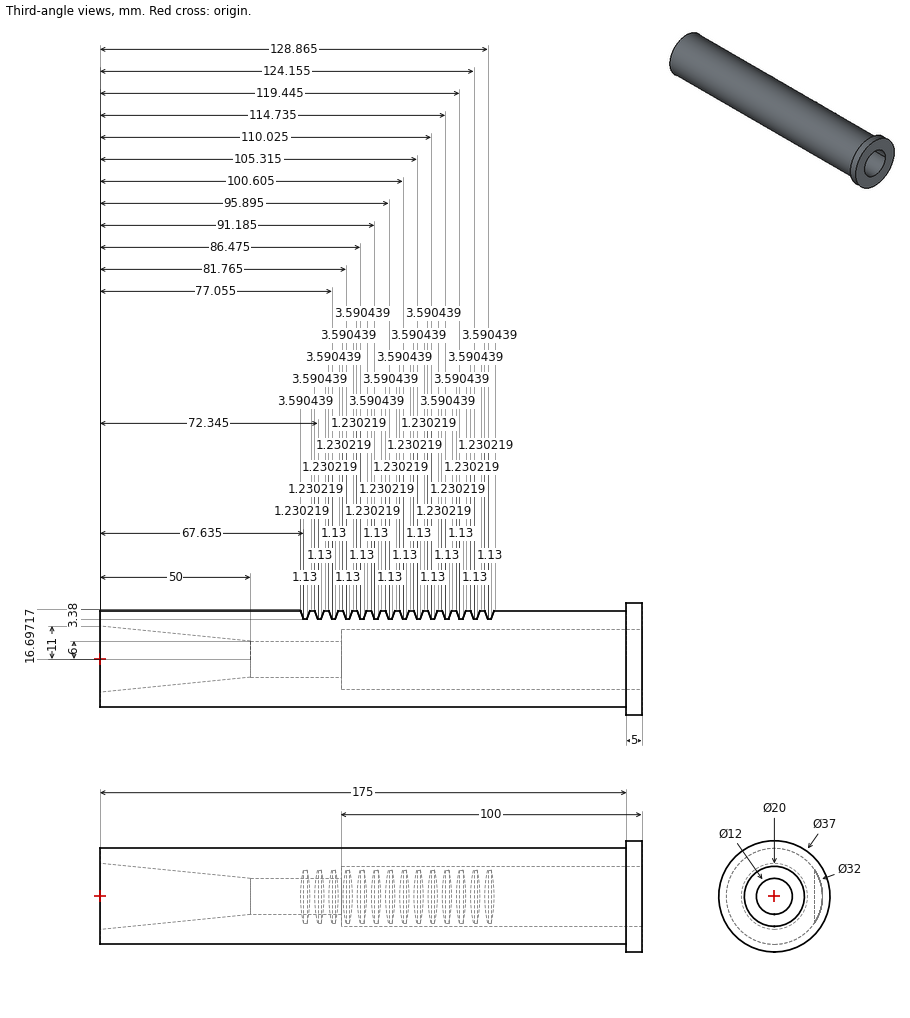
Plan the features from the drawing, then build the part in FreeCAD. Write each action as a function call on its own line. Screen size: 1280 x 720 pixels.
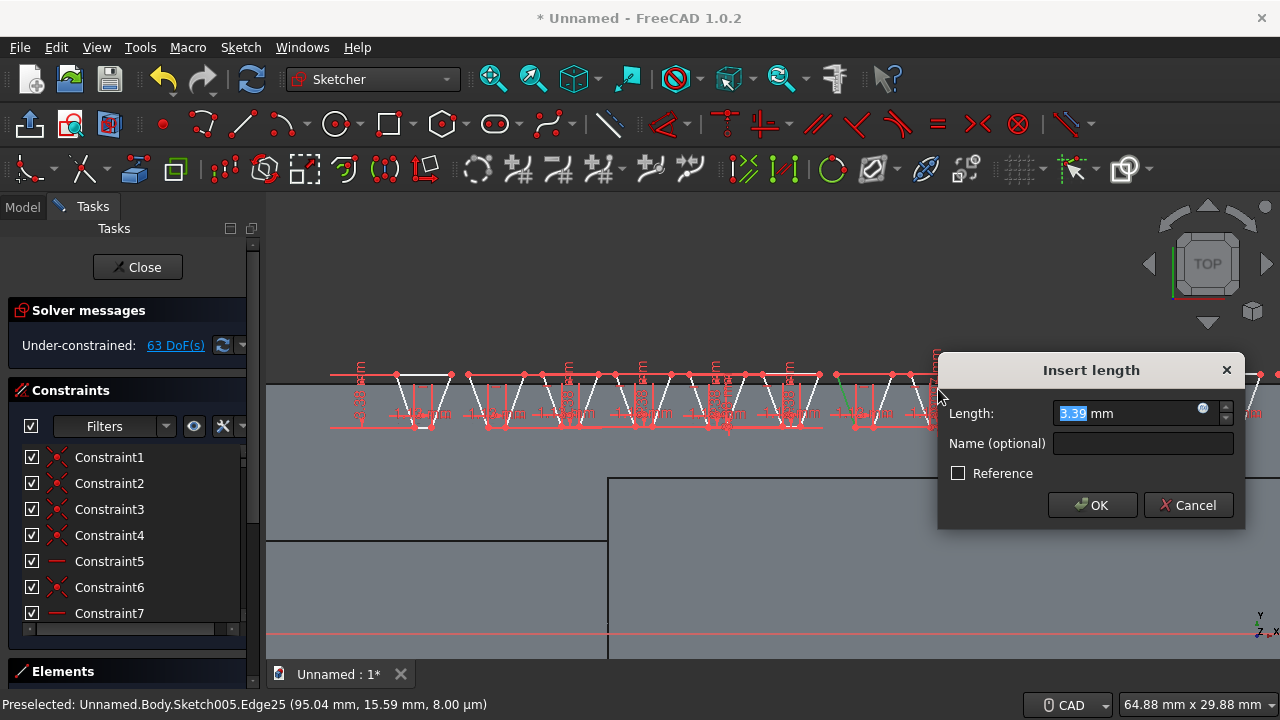
text(3.38)
key(Return)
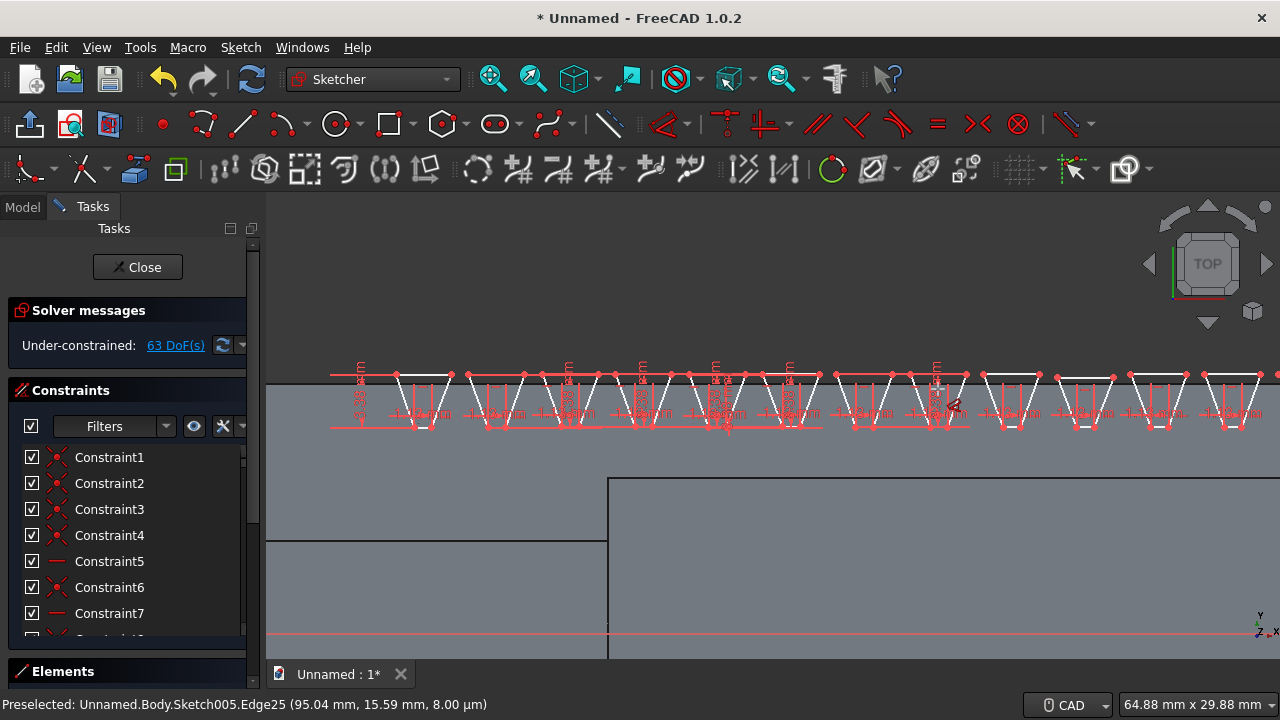
click(916, 390)
click(1012, 389)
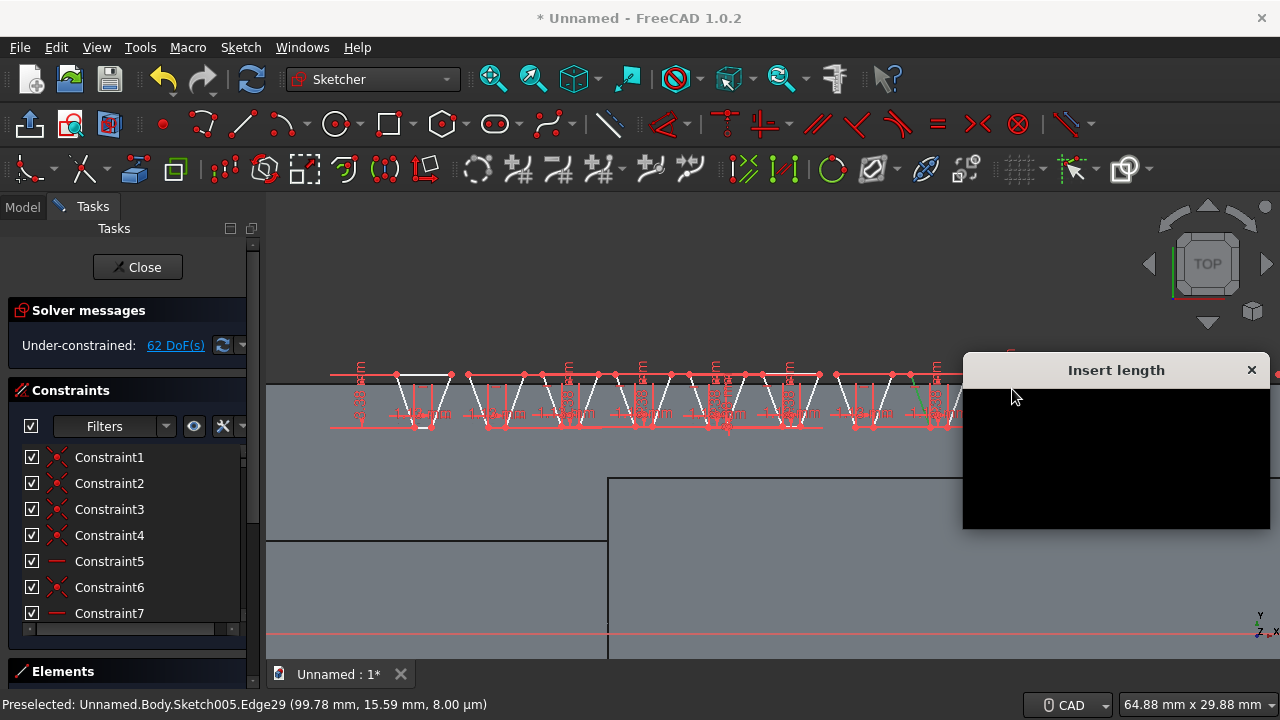
text(3.38)
key(Return)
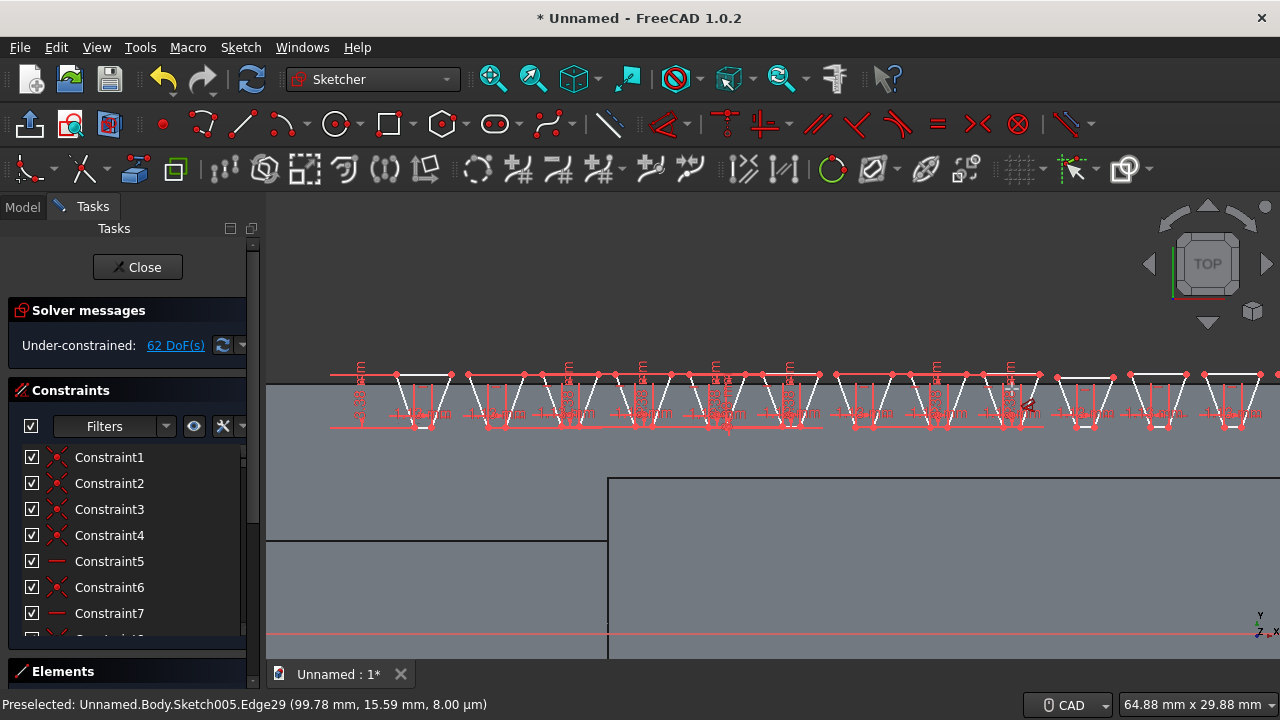
click(989, 390)
click(950, 401)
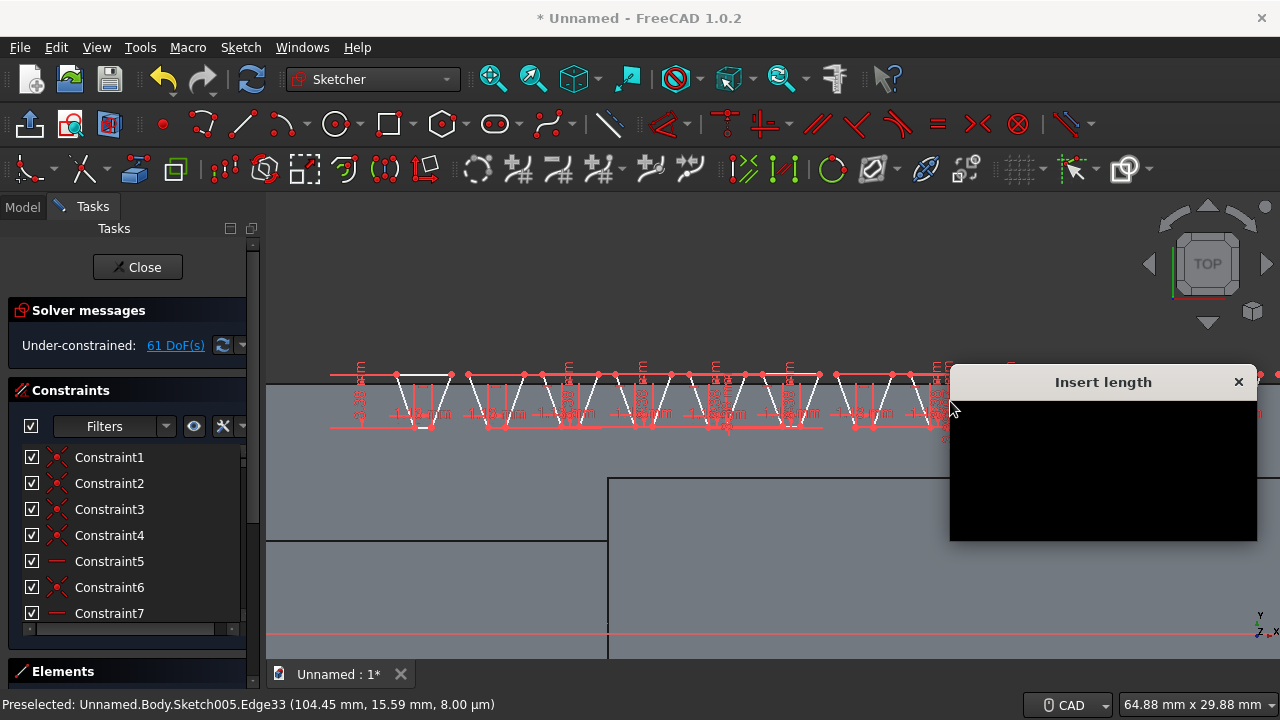
text(3.38)
key(Return)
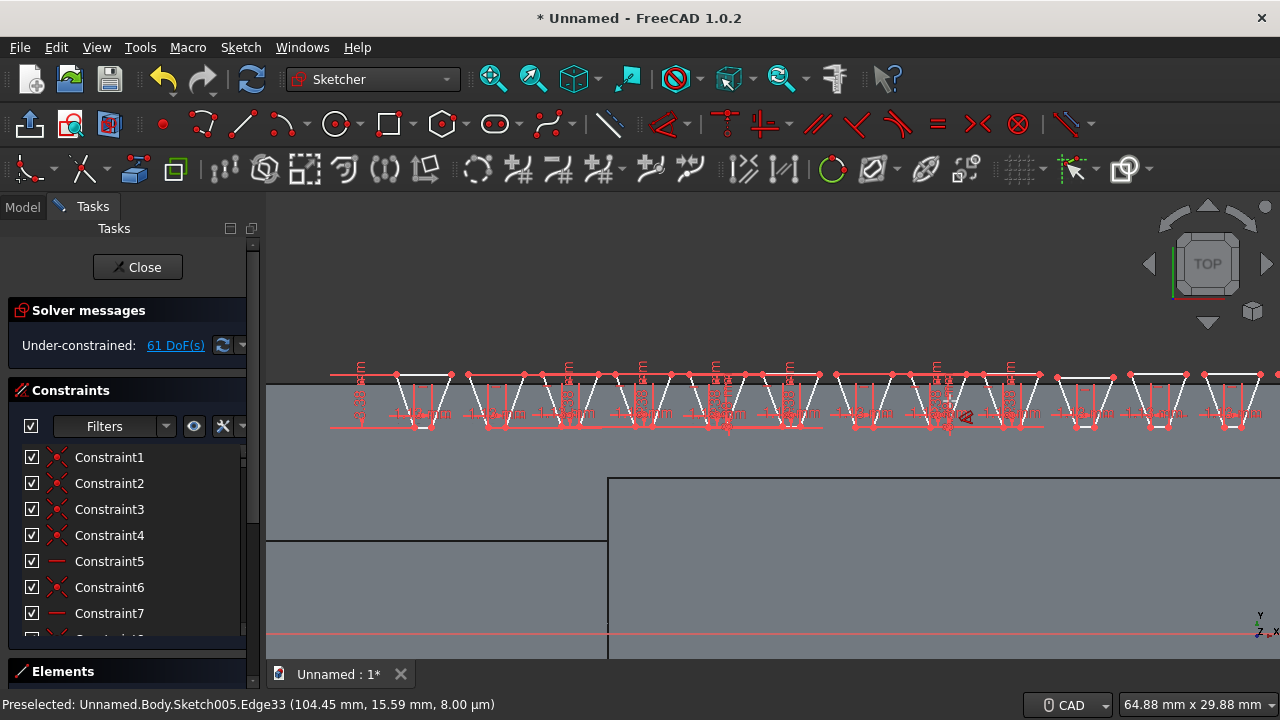
click(1063, 393)
click(976, 414)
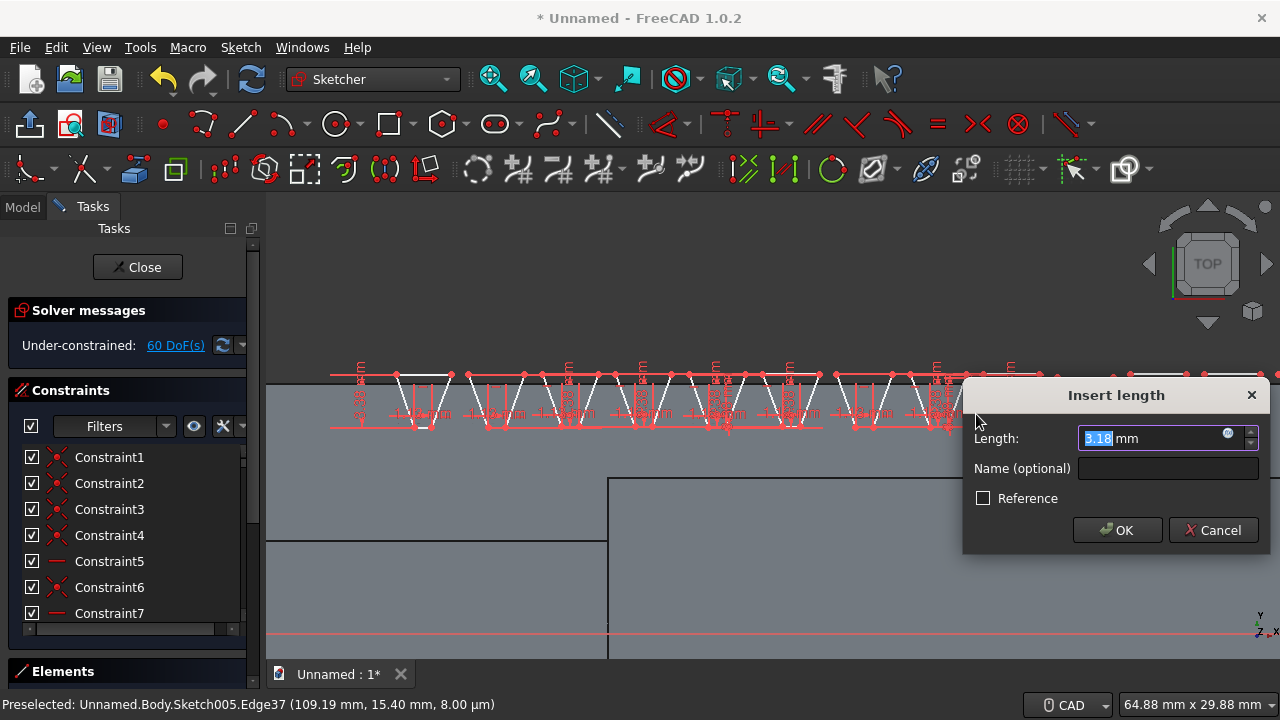
text(3.38)
key(Return)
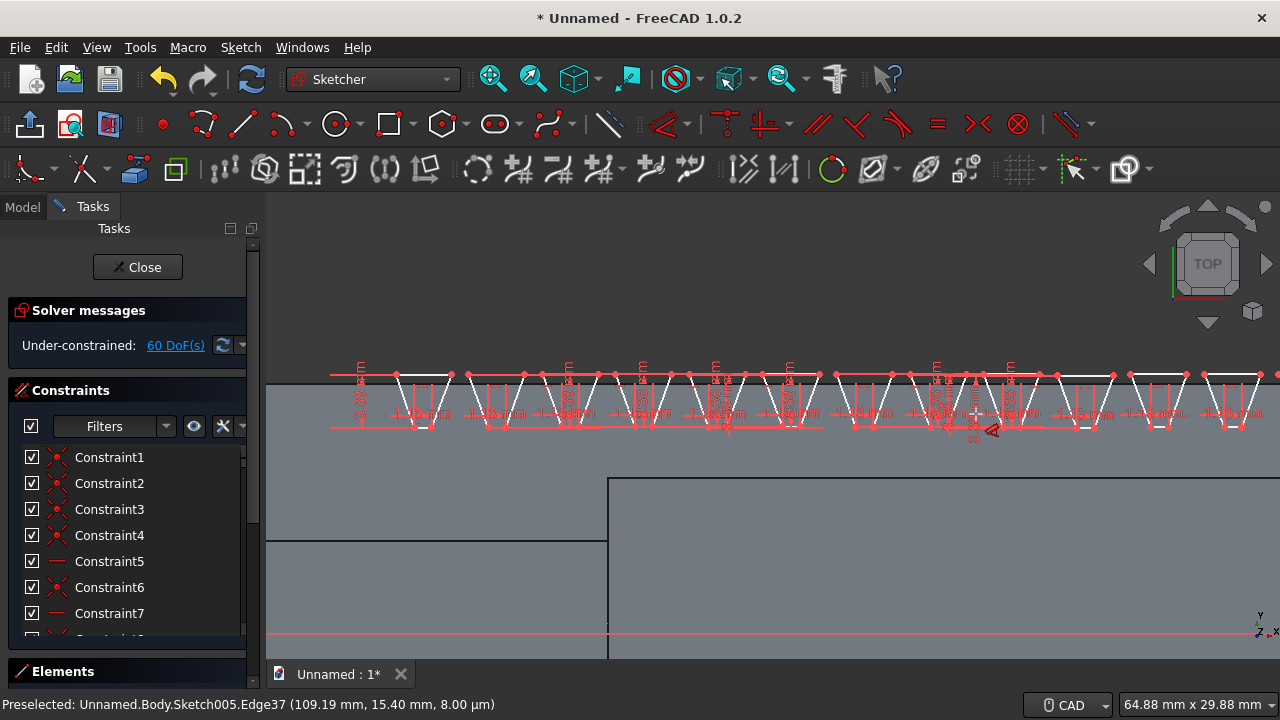
scroll(843, 392, down, 6)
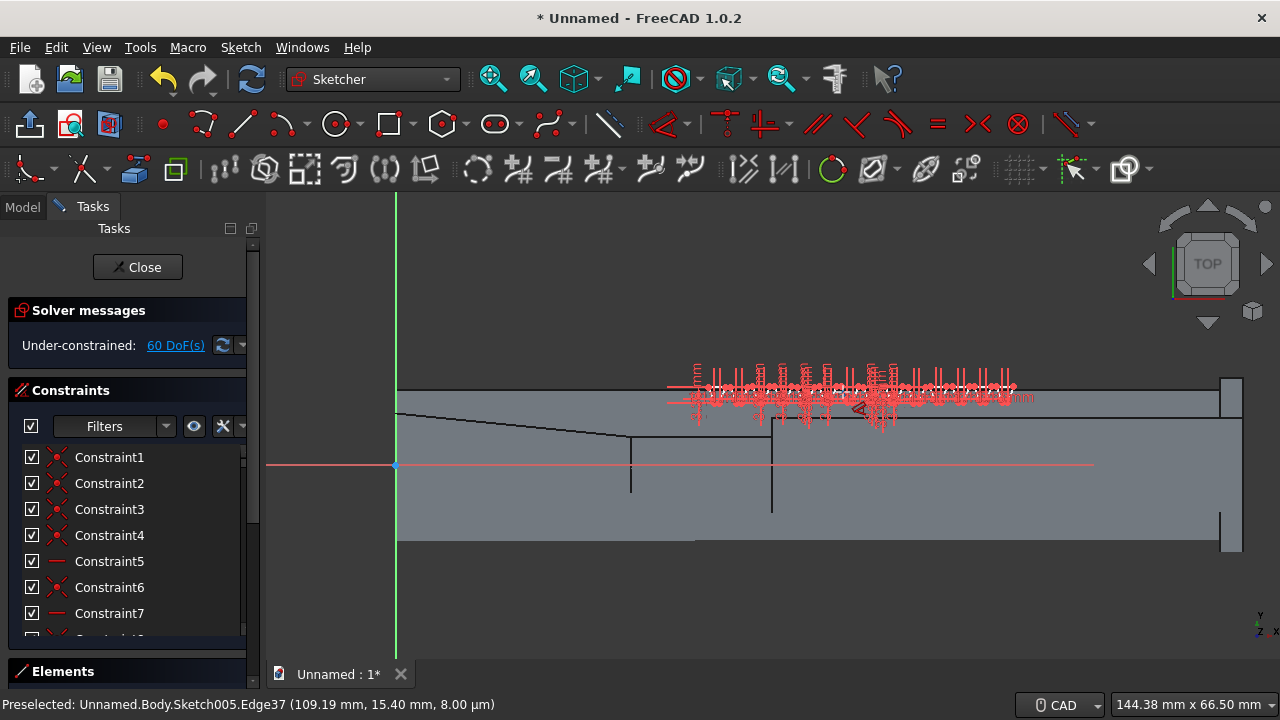
scroll(932, 392, up, 6)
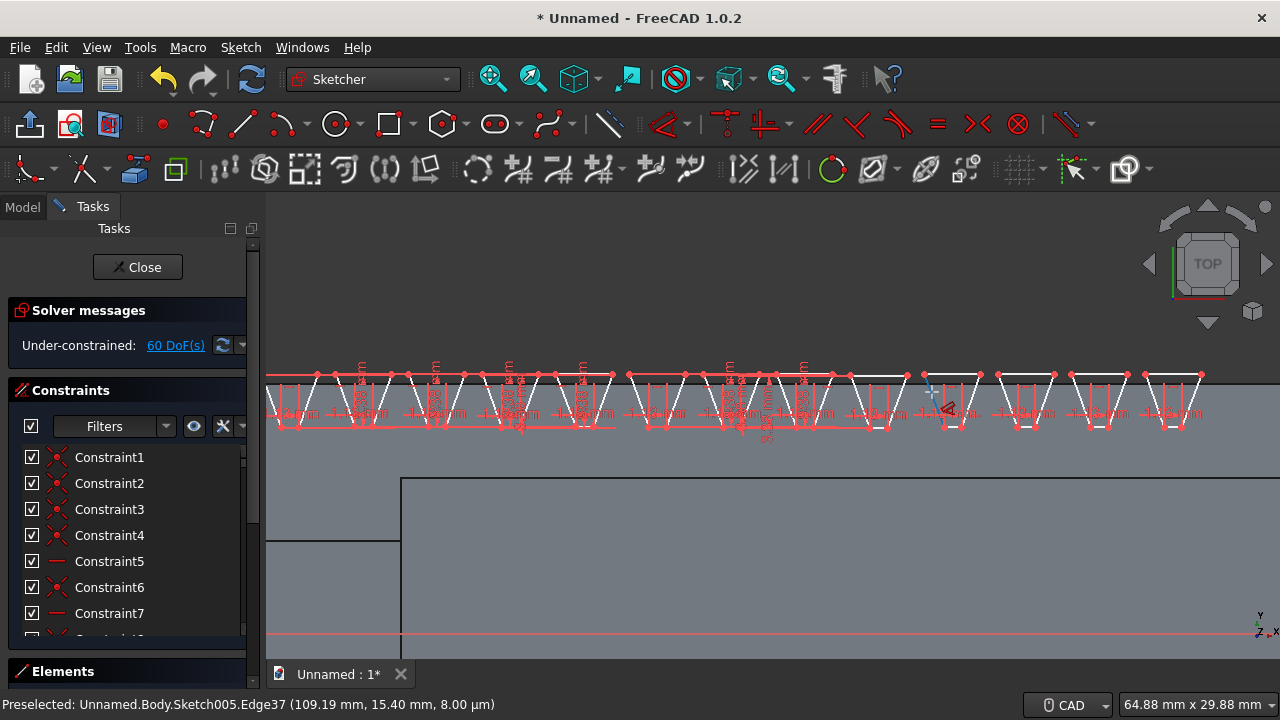
click(930, 390)
click(1026, 389)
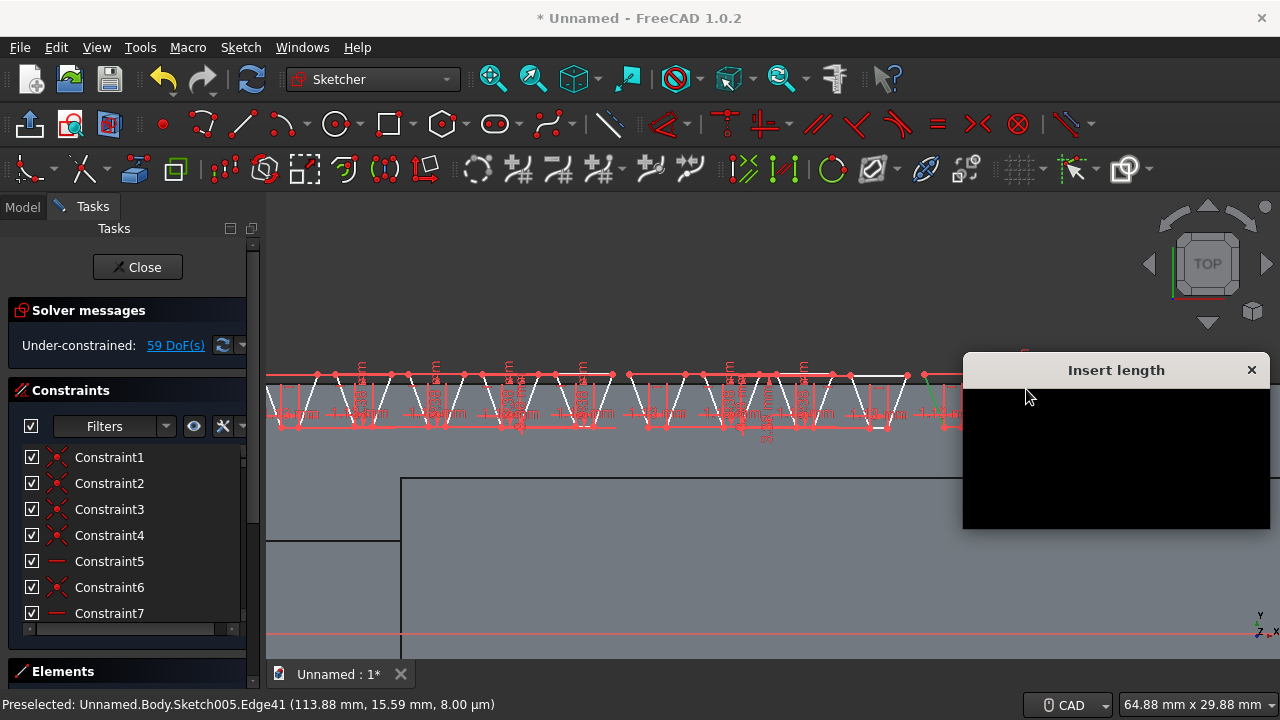
text(3.38)
key(Return)